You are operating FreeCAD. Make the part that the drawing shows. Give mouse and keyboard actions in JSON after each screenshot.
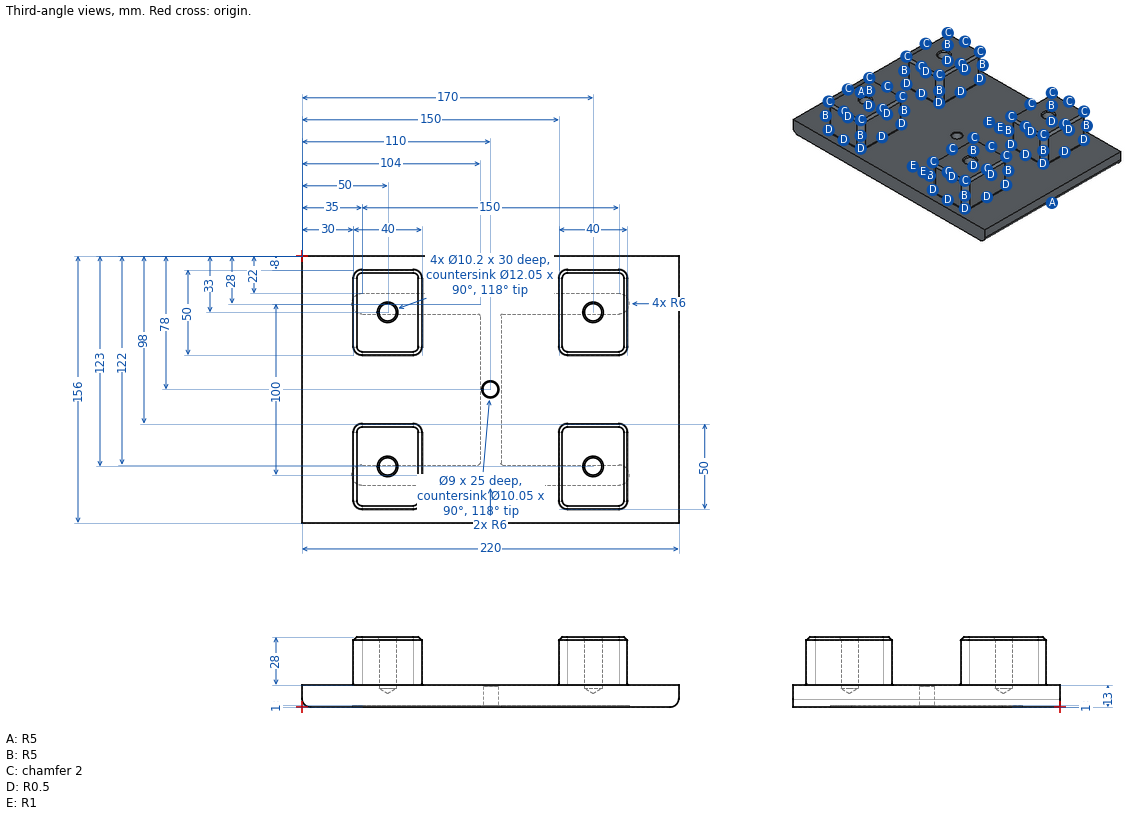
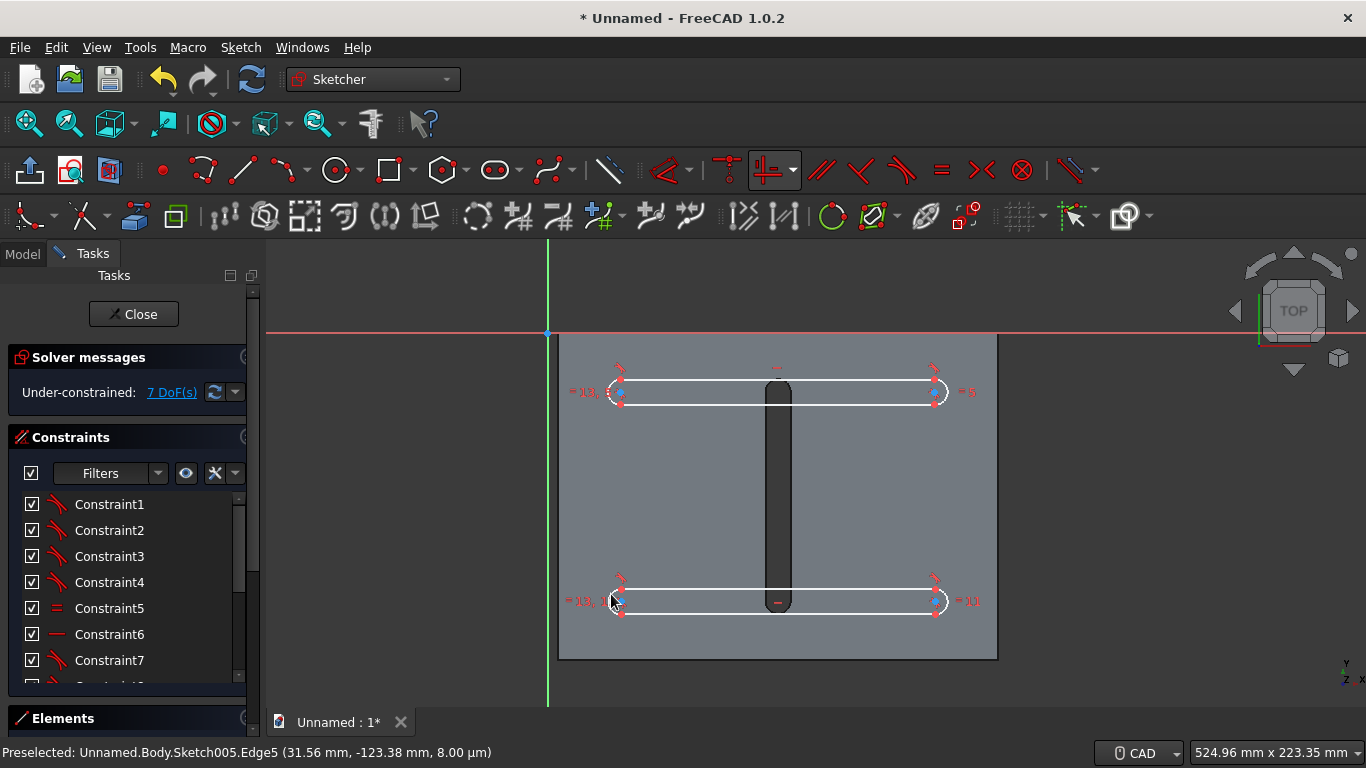
{"action": "left_click", "coordinate": [664, 170]}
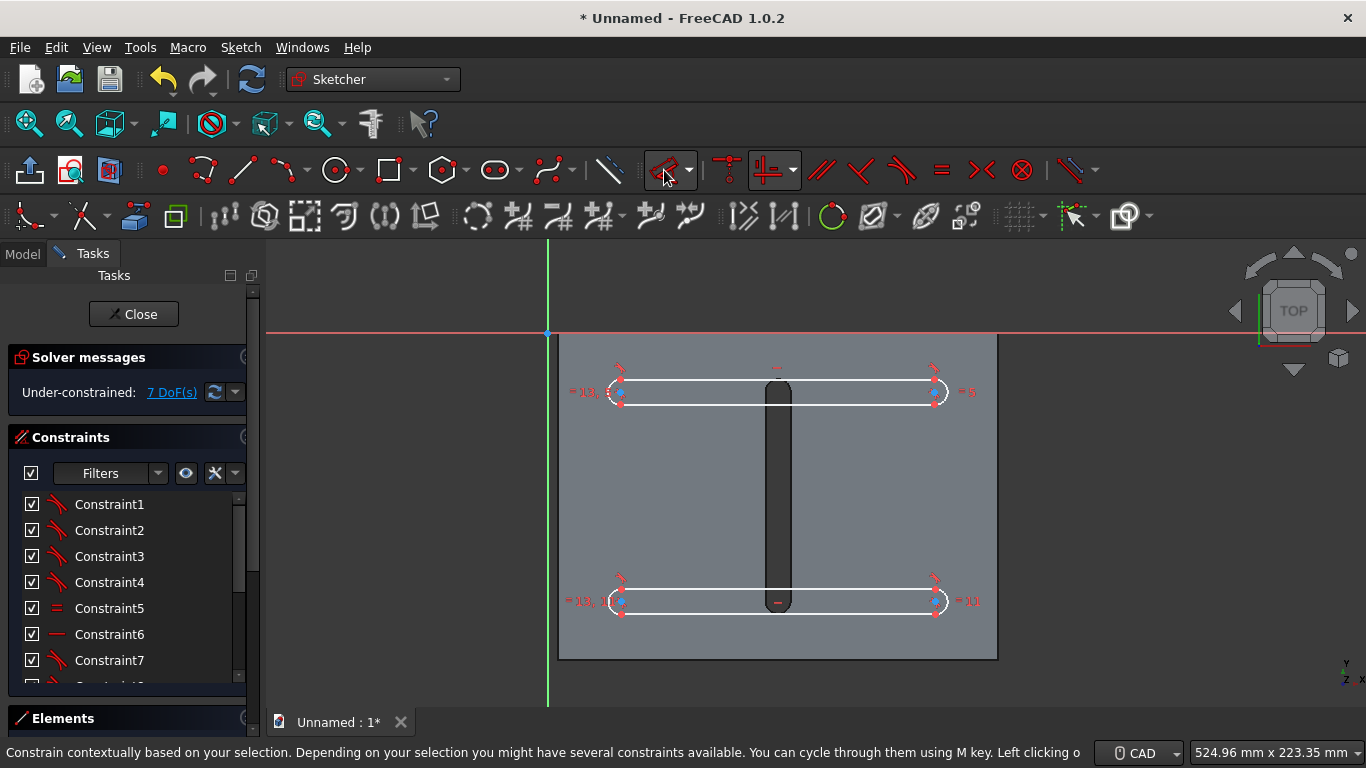
{"action": "scroll", "coordinate": [611, 385], "scroll_direction": "up", "scroll_amount": 6}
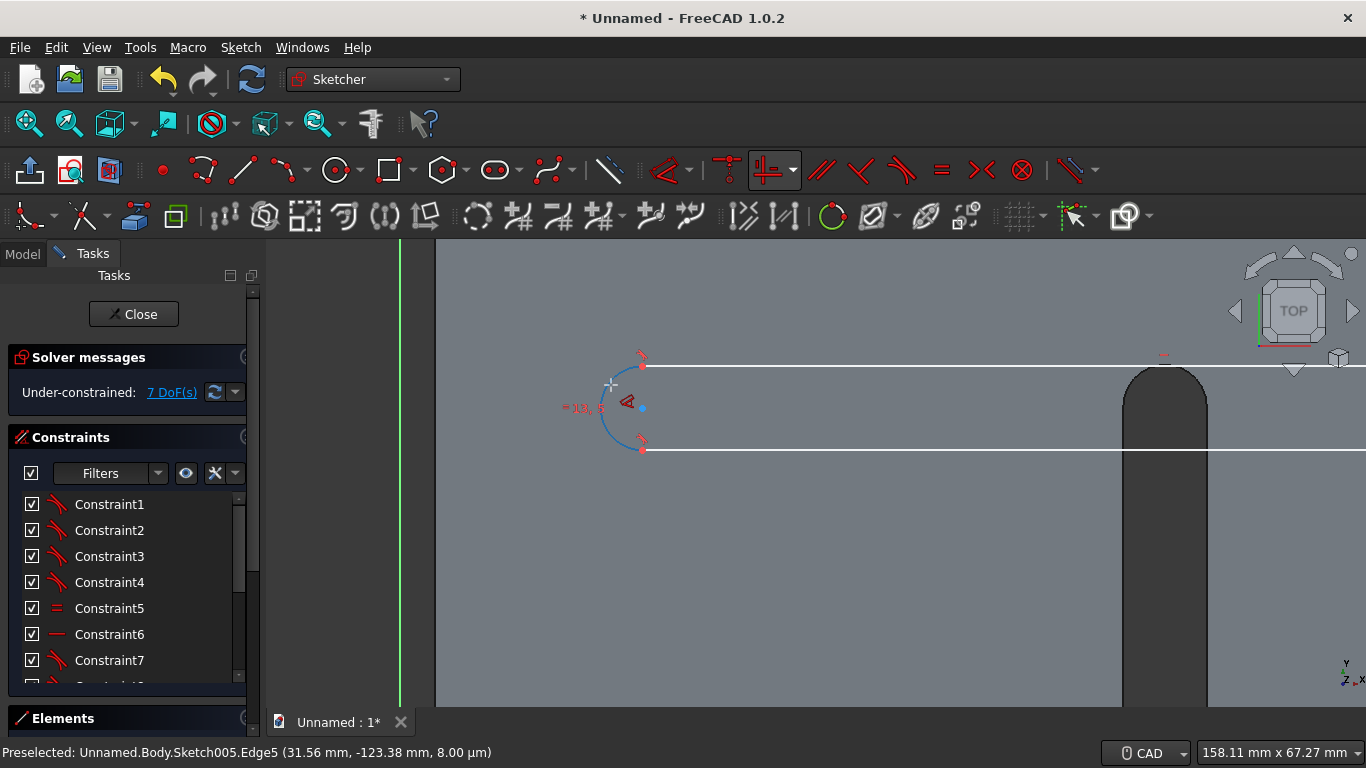
{"action": "left_click", "coordinate": [609, 384]}
{"action": "left_click", "coordinate": [583, 365]}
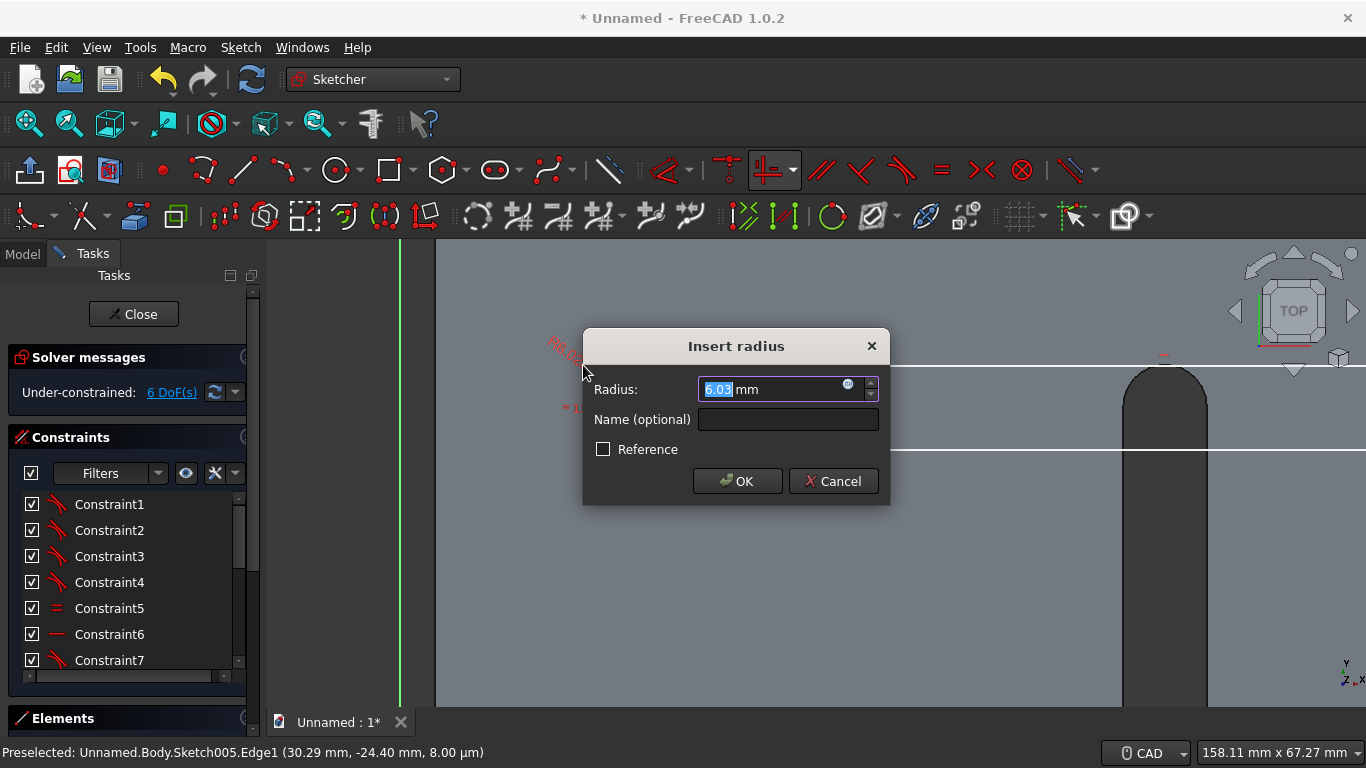
{"action": "type", "text": "6"}
{"action": "key", "text": "Return"}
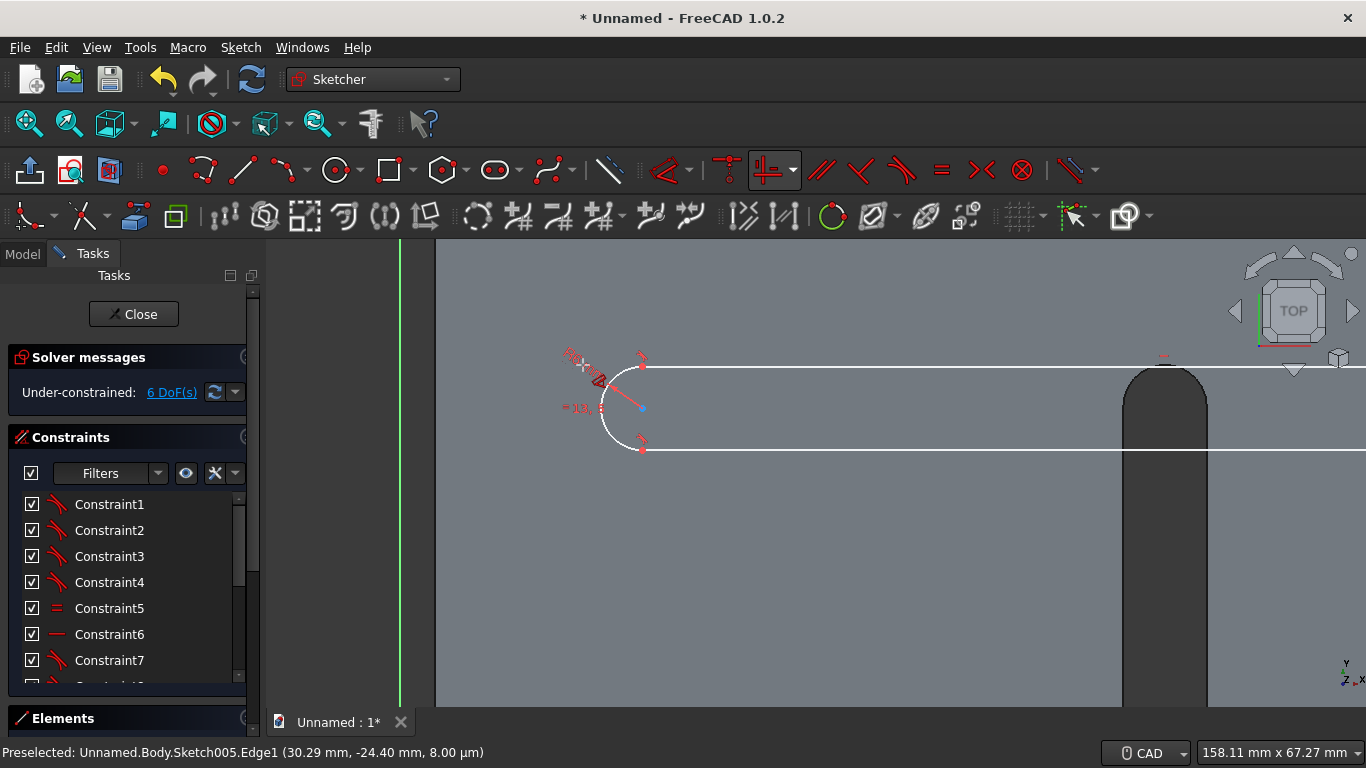
{"action": "scroll", "coordinate": [611, 385], "scroll_direction": "down", "scroll_amount": 6}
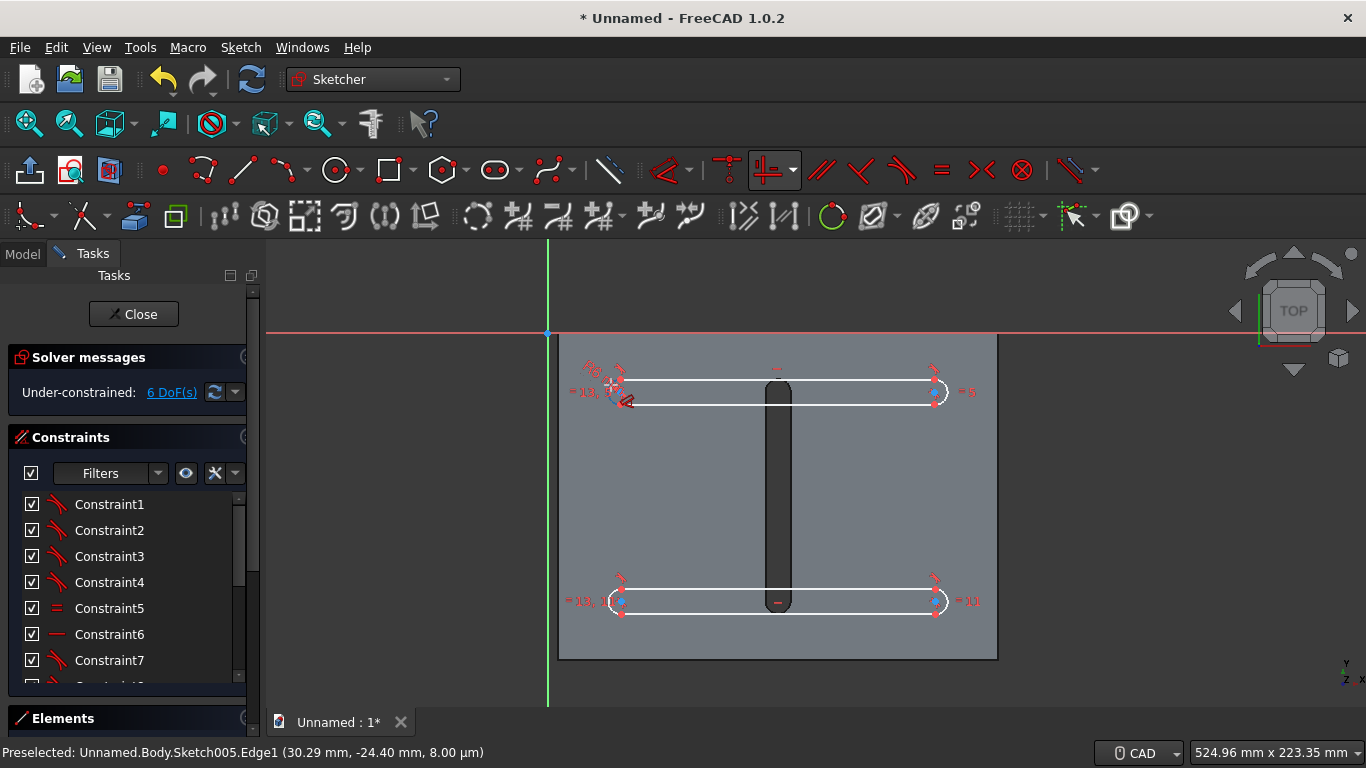
{"action": "left_click", "coordinate": [715, 380]}
{"action": "left_click", "coordinate": [778, 438]}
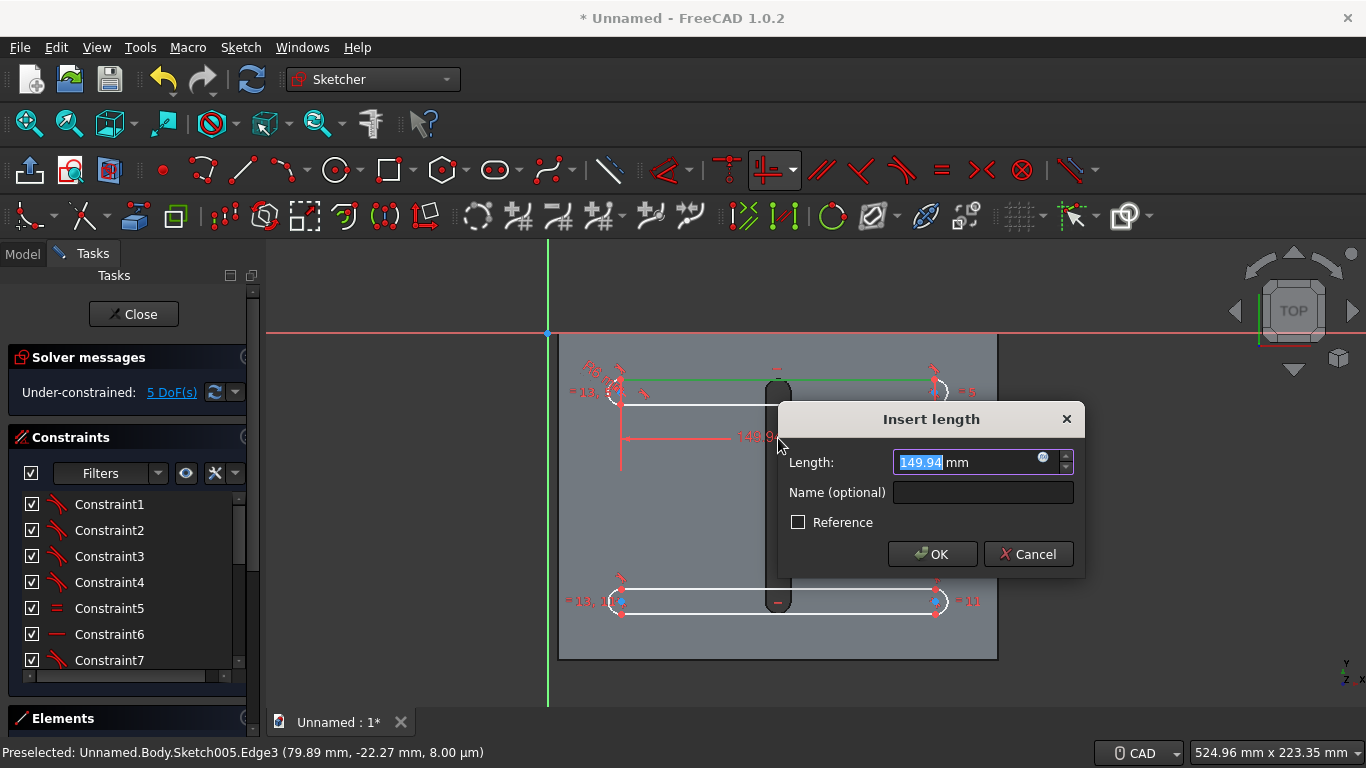
{"action": "type", "text": "150"}
{"action": "key", "text": "Return"}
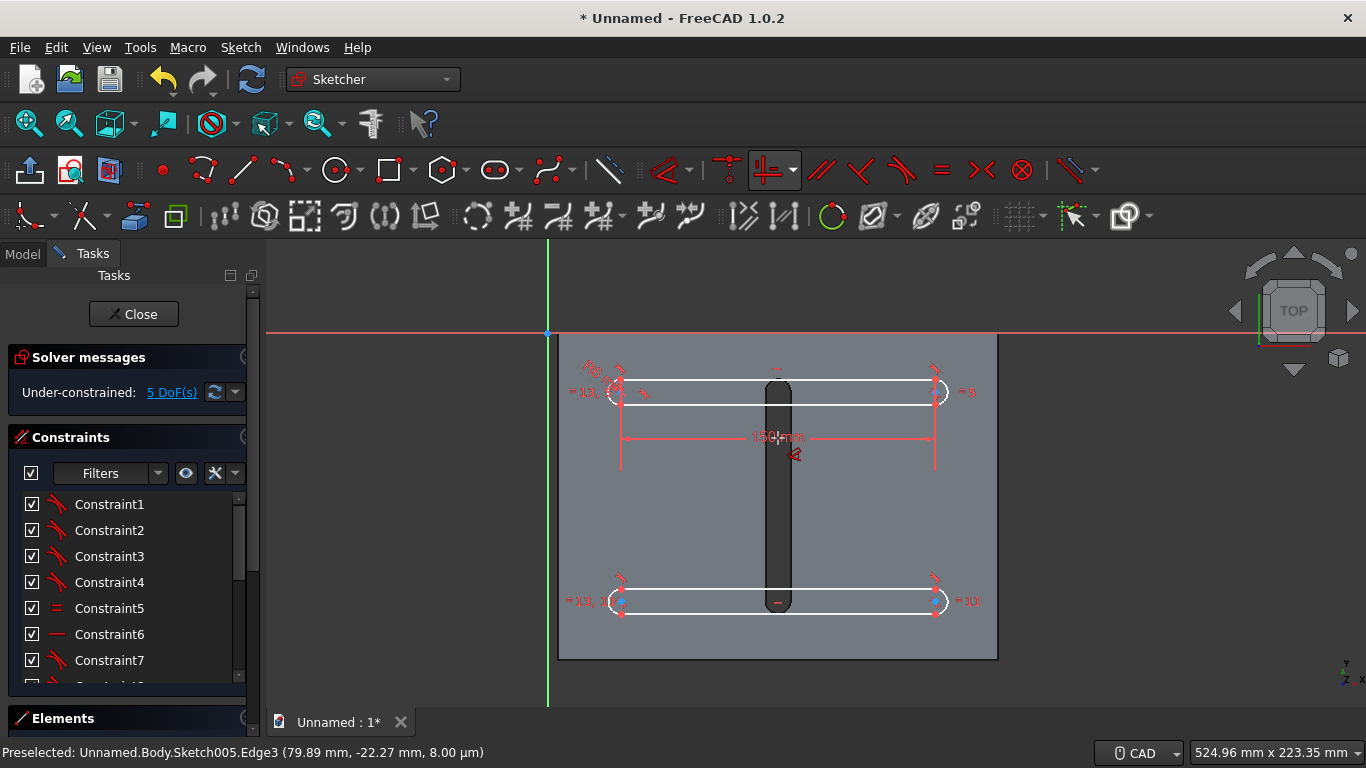
{"action": "left_click", "coordinate": [715, 589]}
{"action": "left_click", "coordinate": [778, 555]}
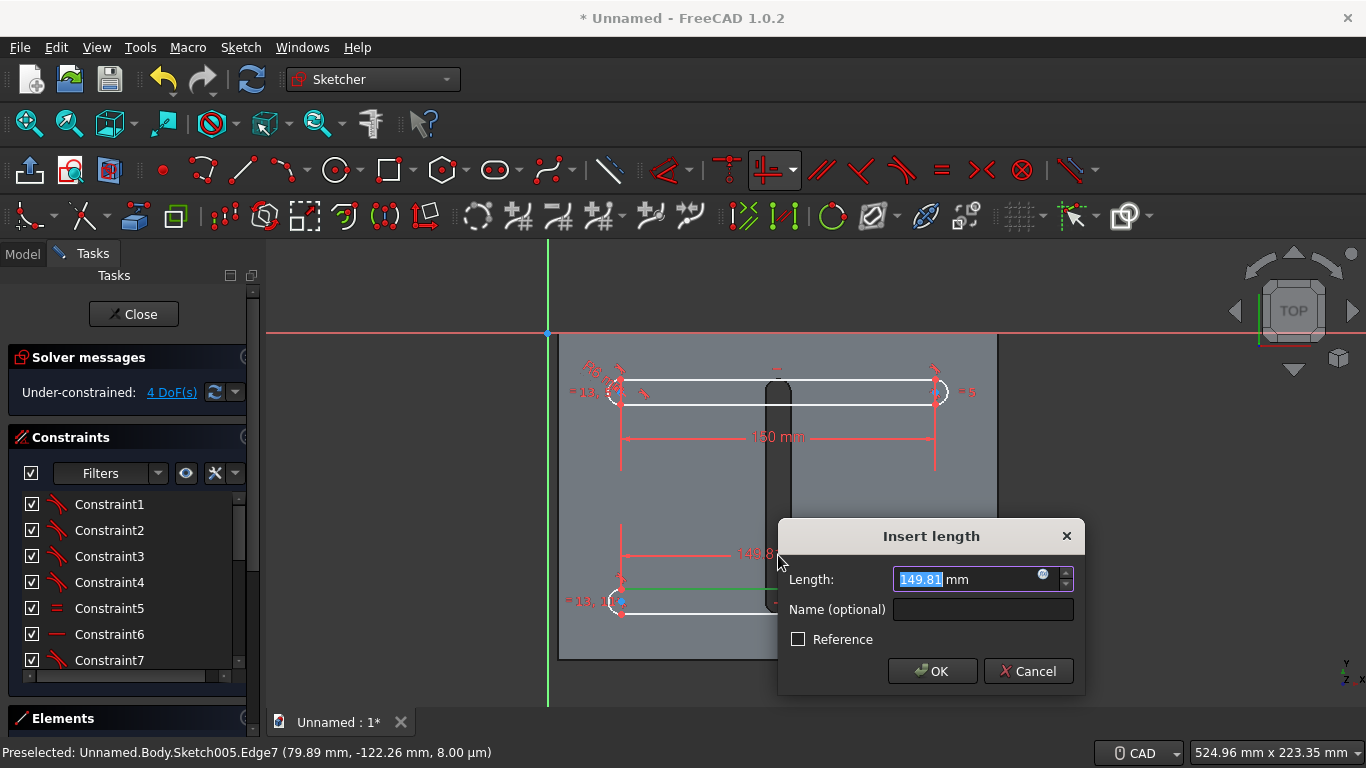
{"action": "type", "text": "150"}
{"action": "key", "text": "Return"}